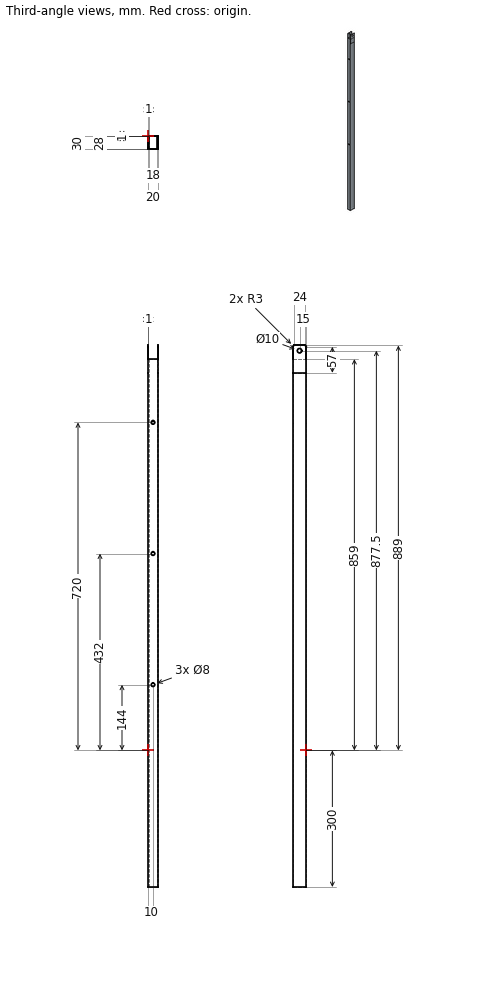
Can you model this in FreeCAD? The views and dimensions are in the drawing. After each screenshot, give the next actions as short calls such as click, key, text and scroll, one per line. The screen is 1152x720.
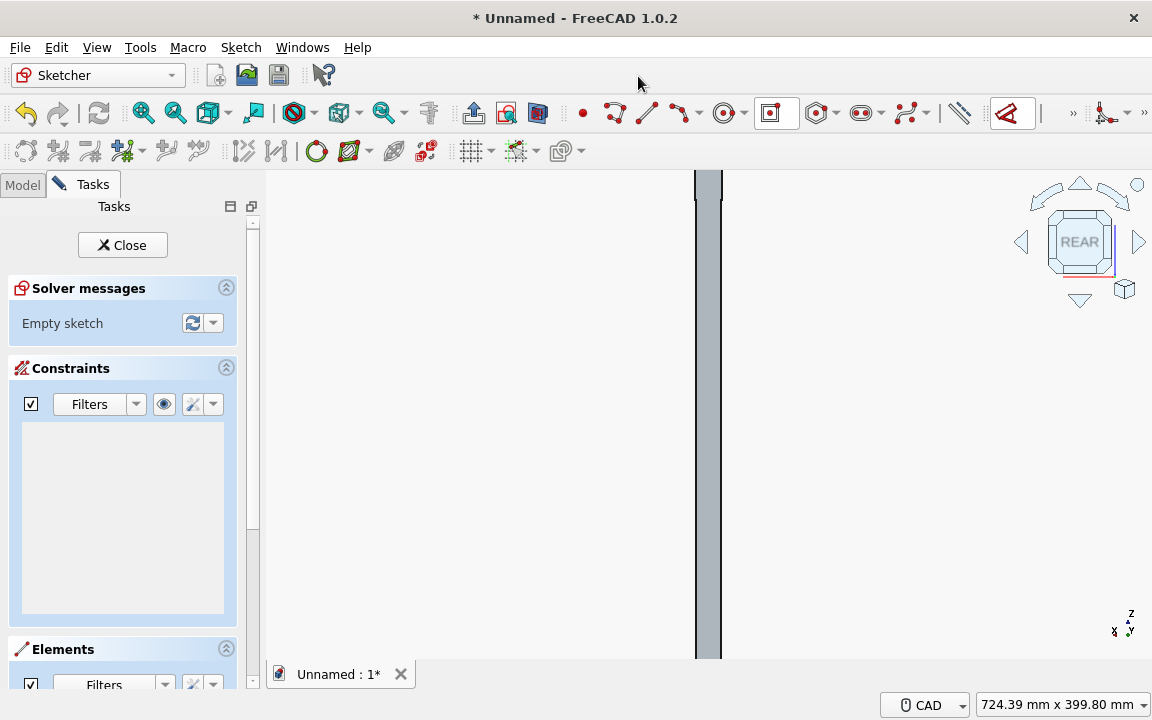
scroll(599, 207, down, 5)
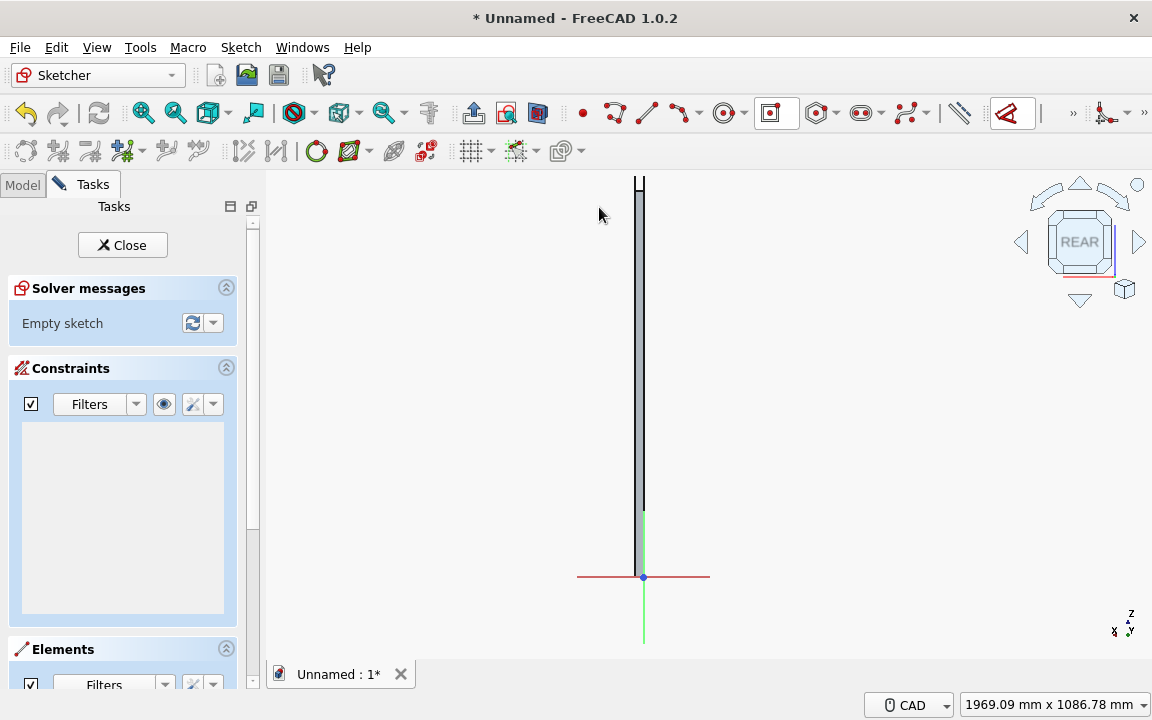
key(g)
key(c)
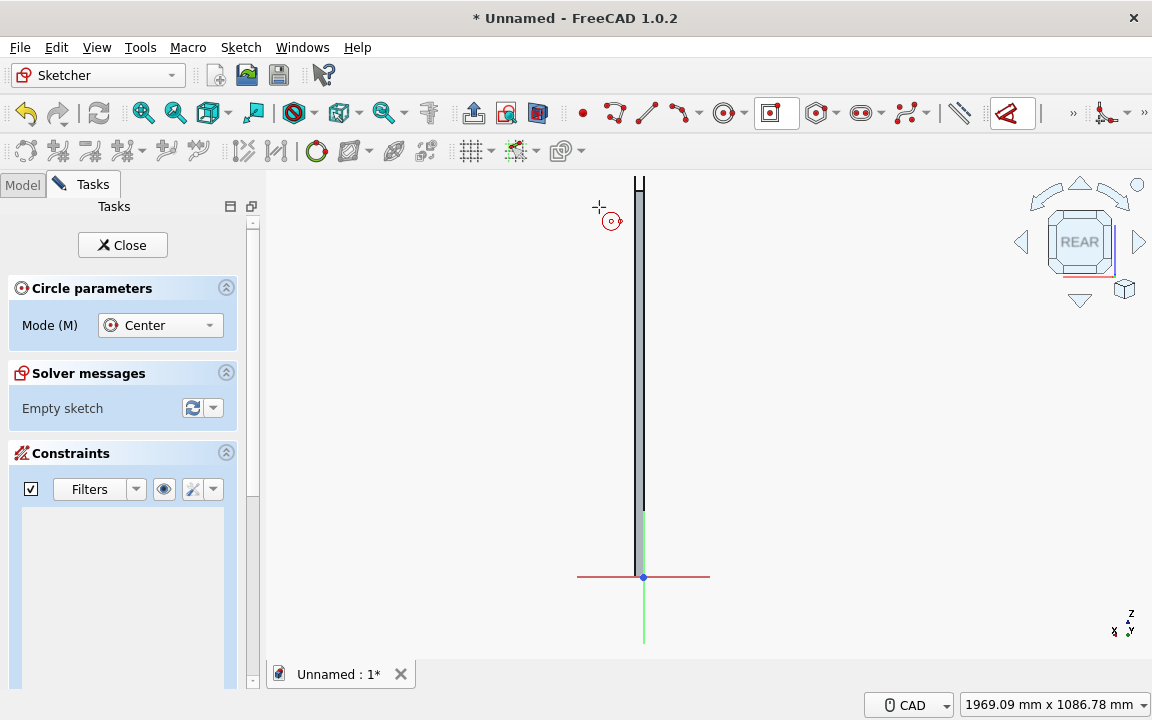
scroll(639, 513, up, 13)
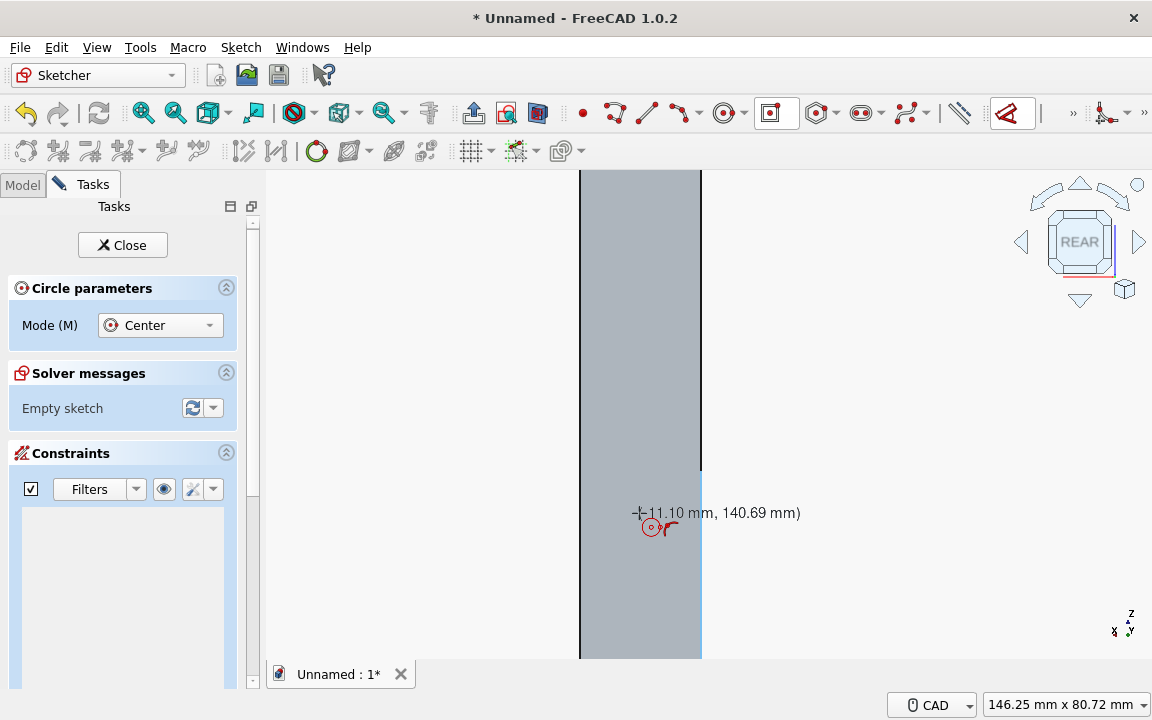
scroll(639, 514, down, 13)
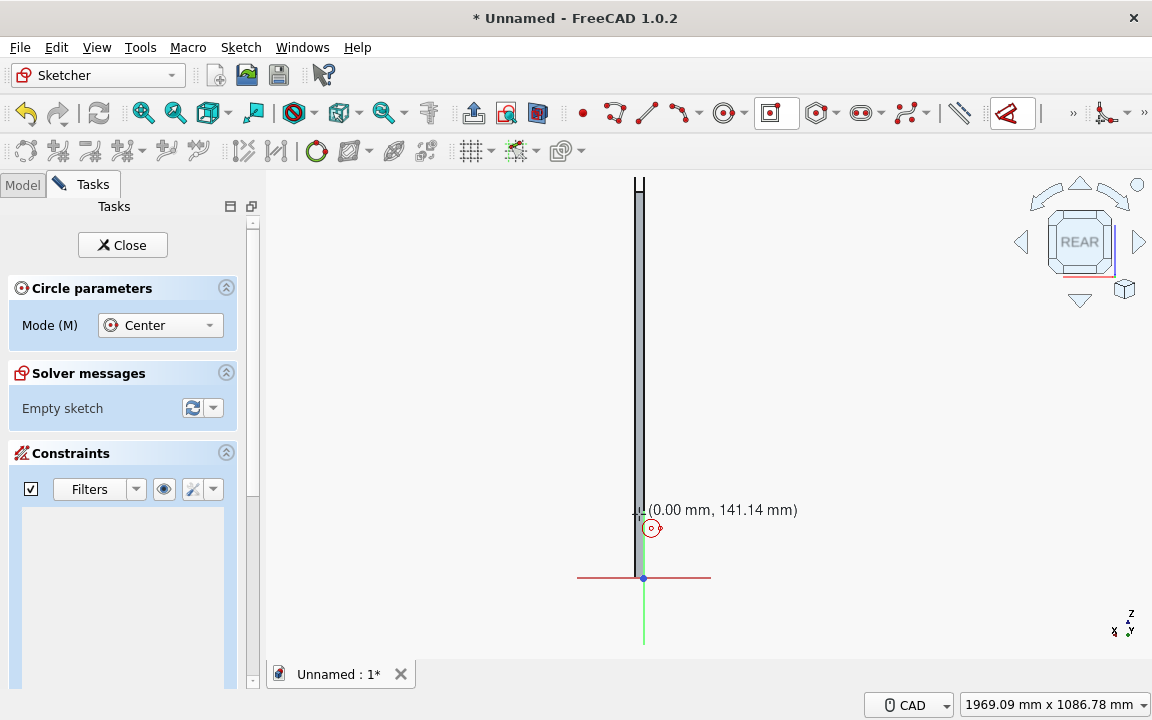
scroll(639, 513, up, 7)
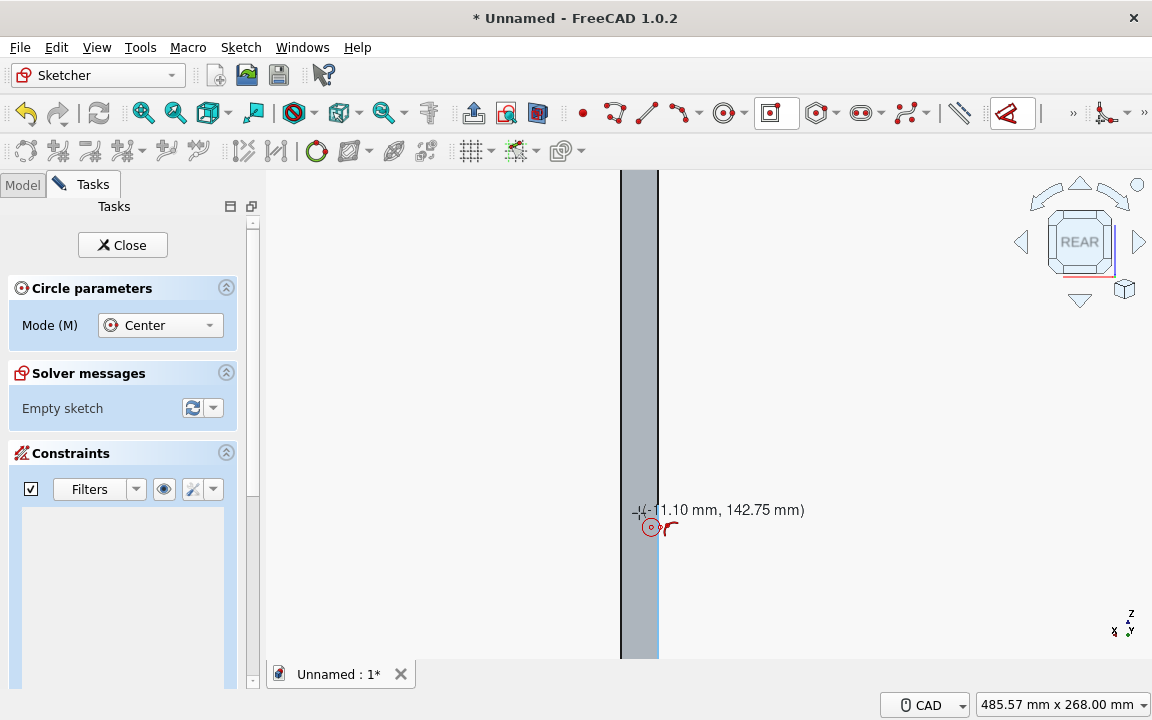
click(640, 513)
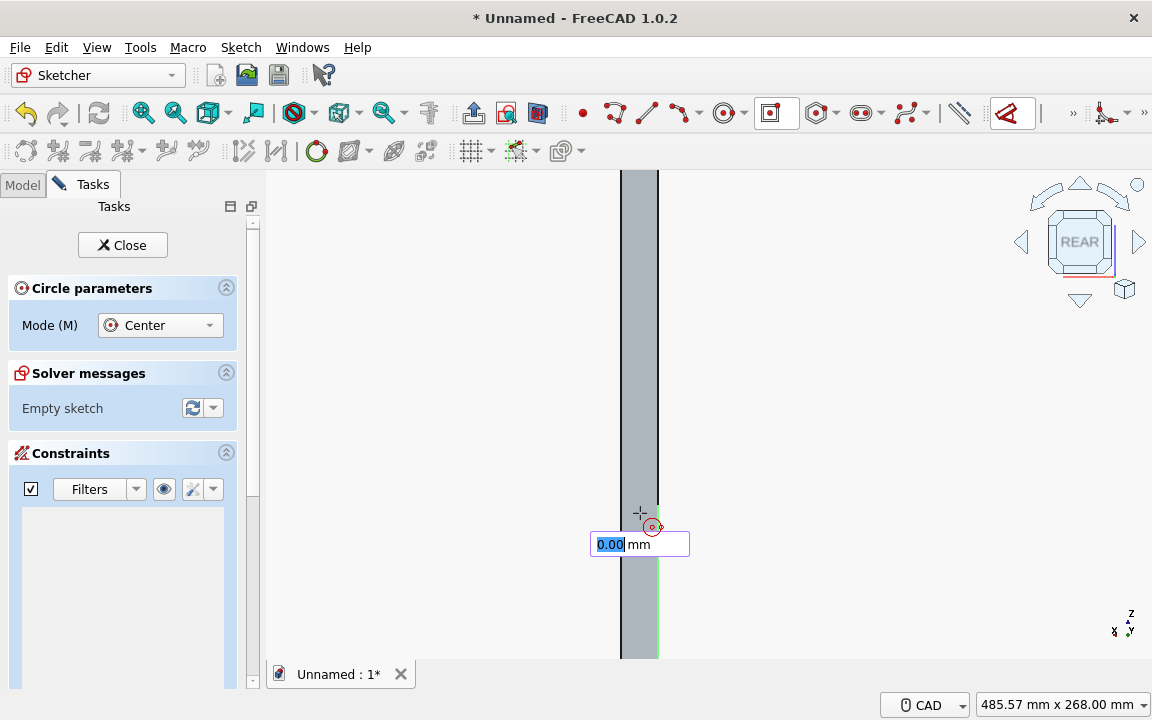
scroll(635, 507, up, 4)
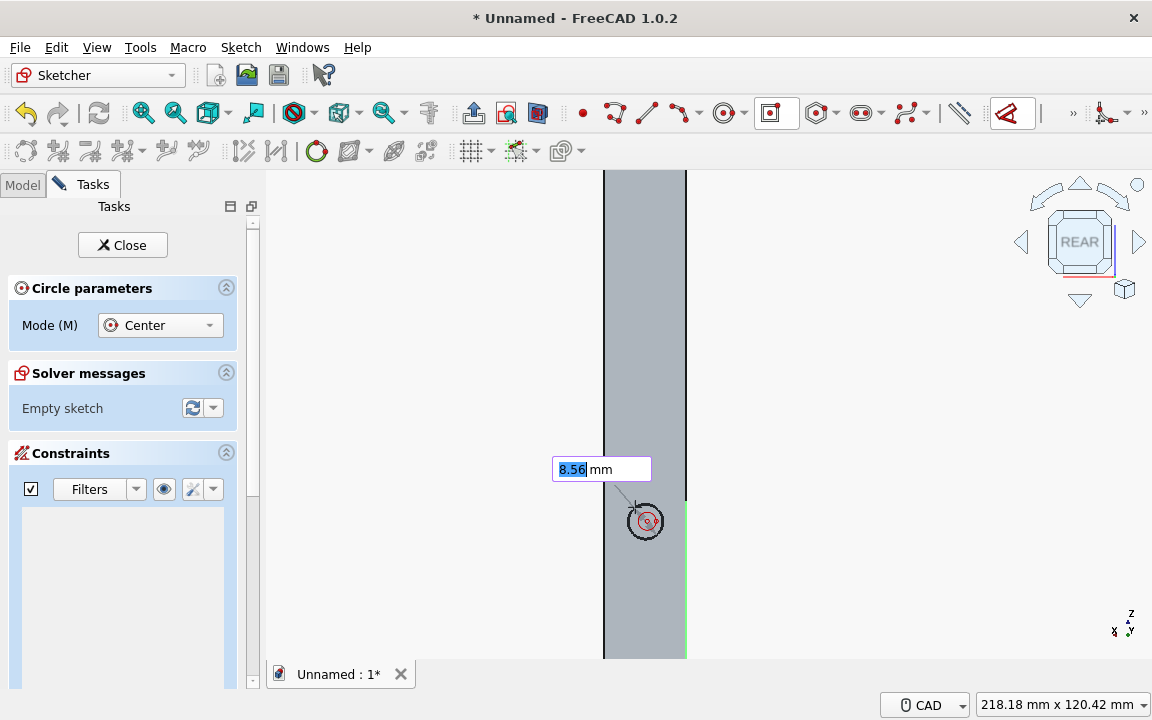
click(634, 507)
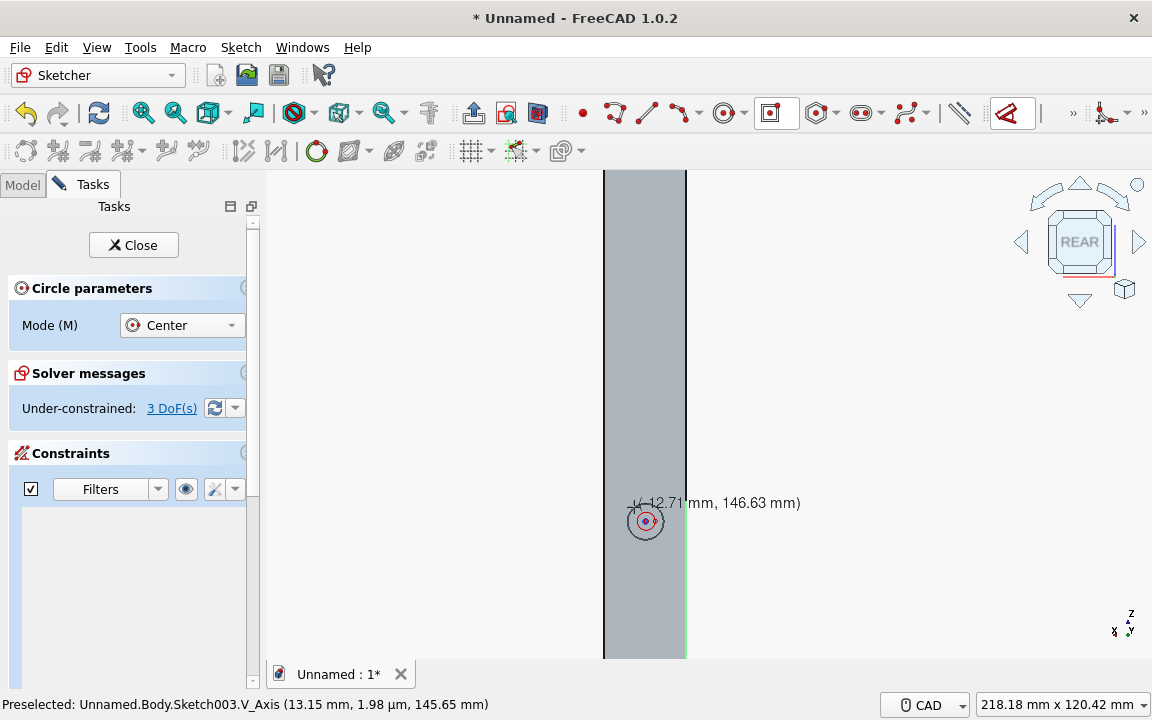
scroll(638, 512, down, 11)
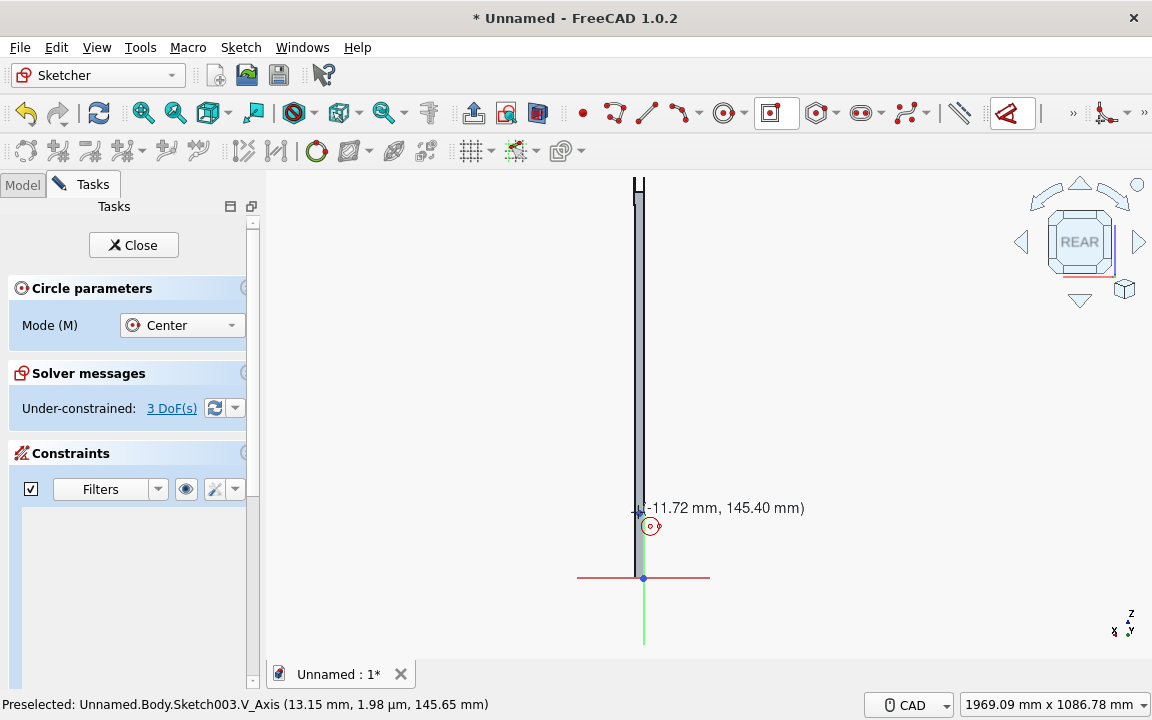
scroll(639, 384, up, 13)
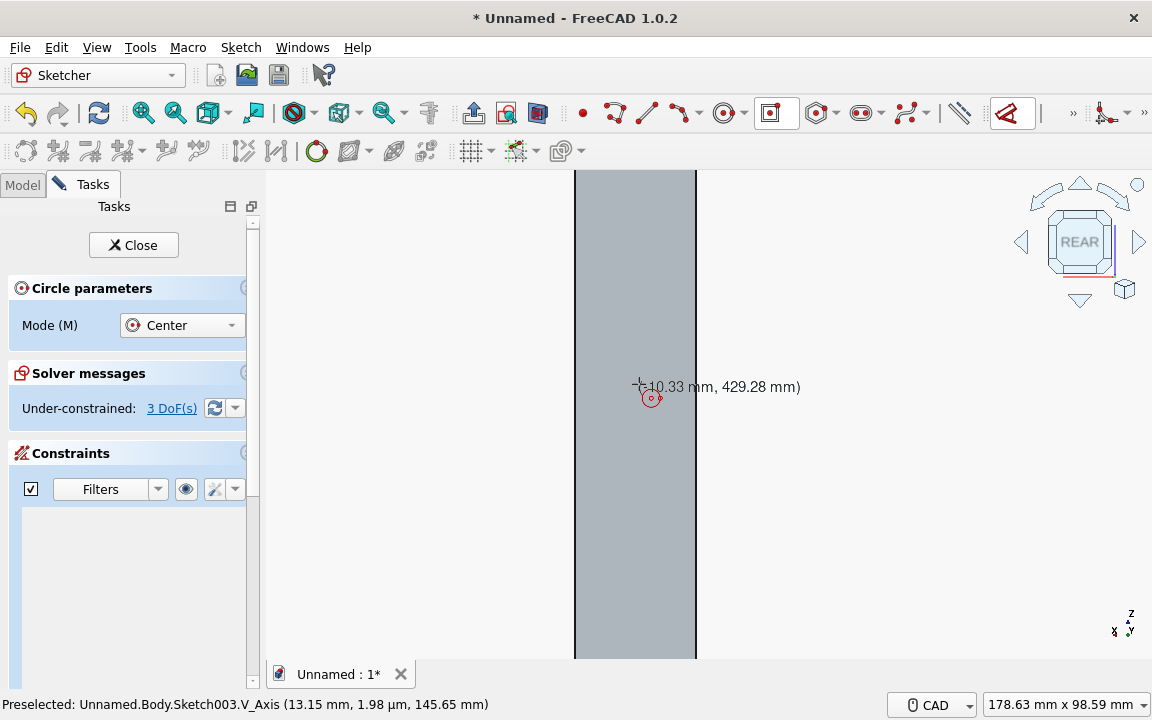
scroll(639, 384, down, 13)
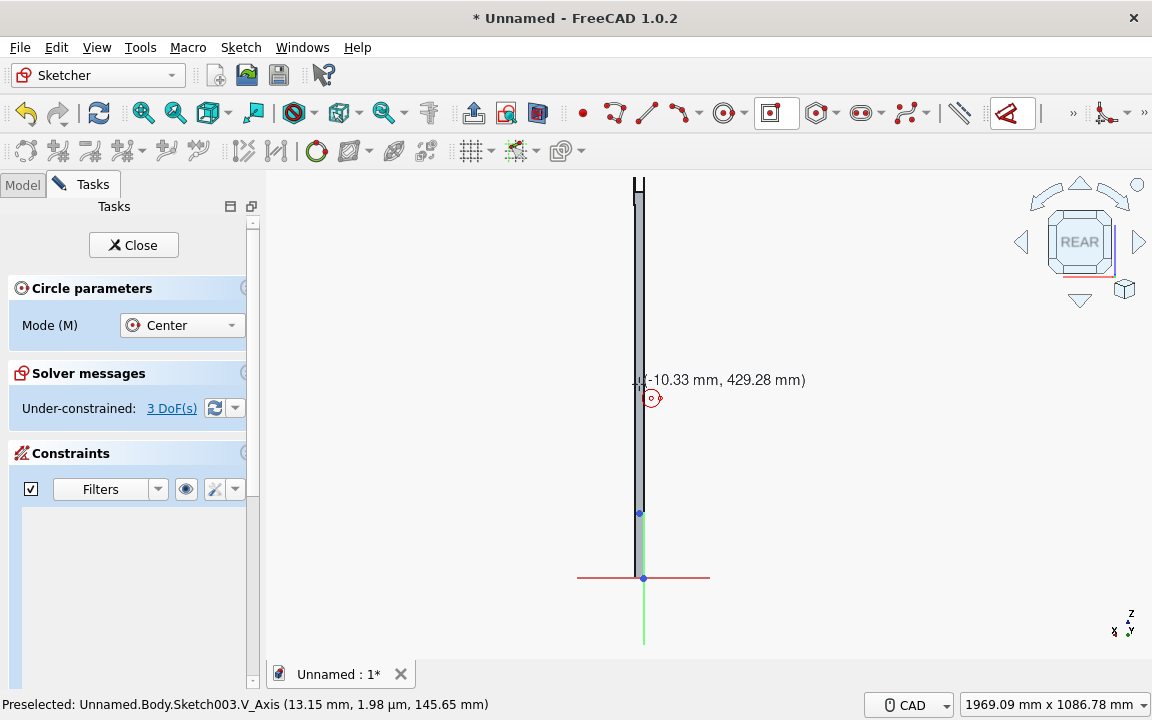
scroll(639, 384, up, 7)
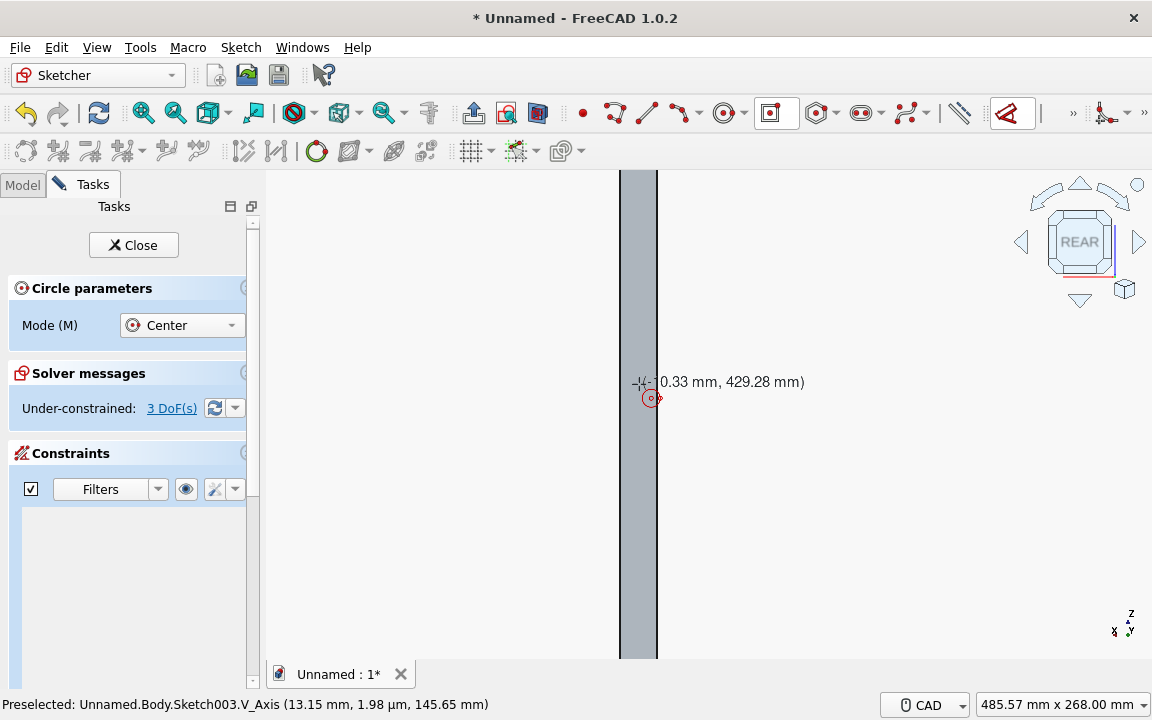
click(638, 382)